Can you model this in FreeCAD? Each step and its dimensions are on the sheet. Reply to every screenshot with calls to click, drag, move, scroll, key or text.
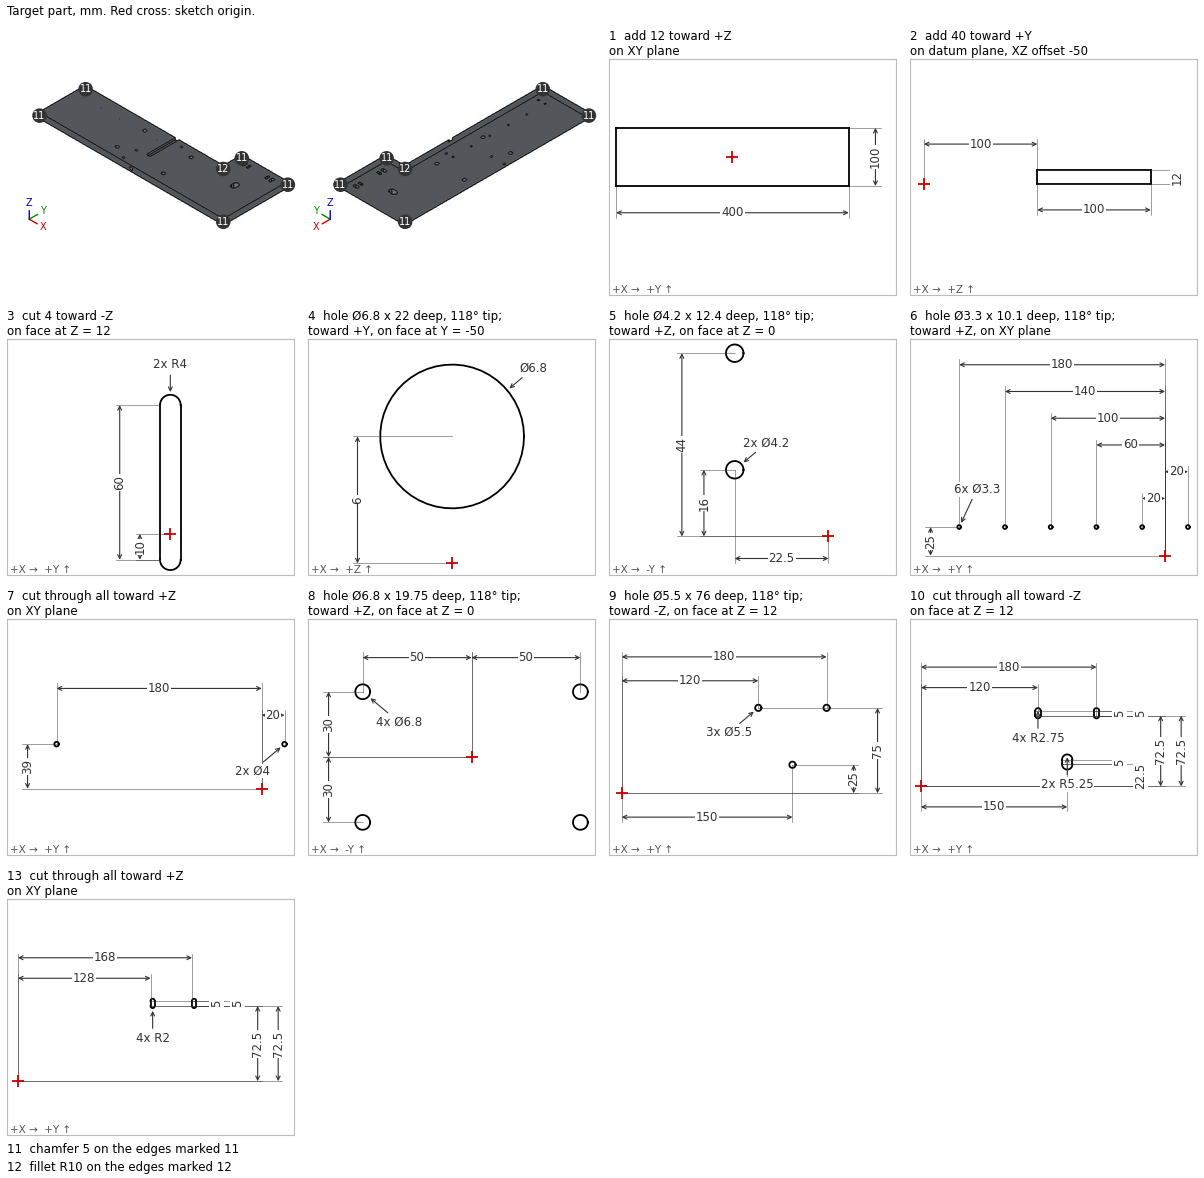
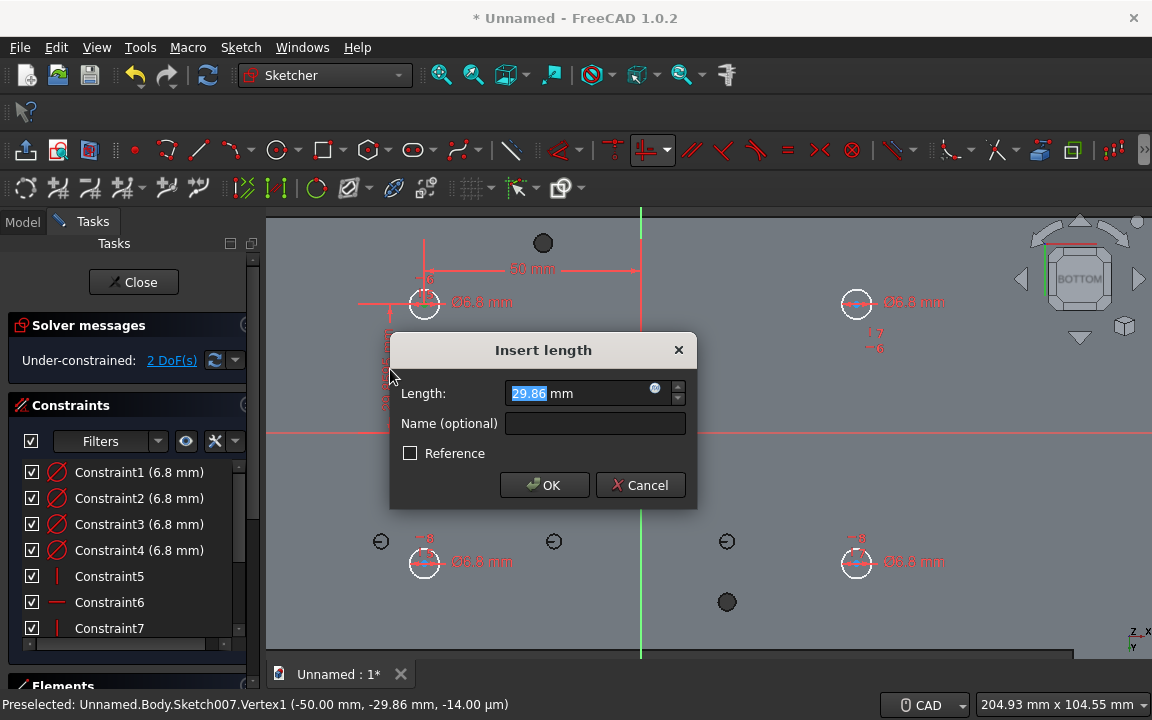
text(30)
key(Return)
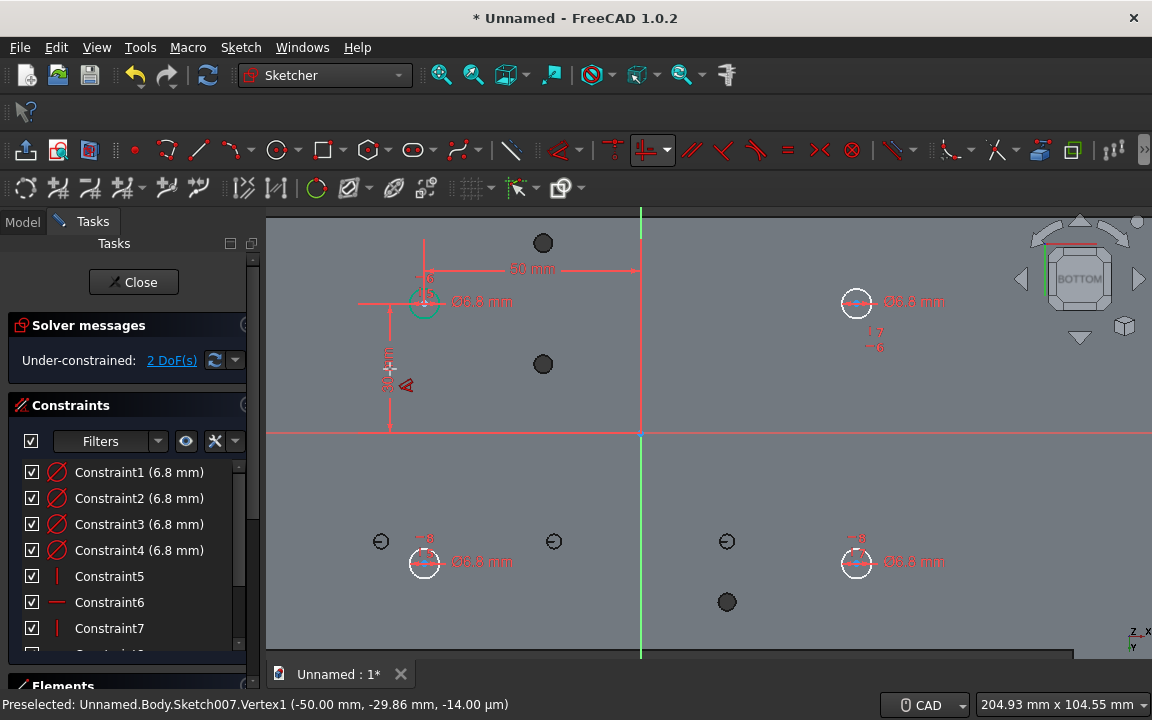
click(424, 564)
click(390, 499)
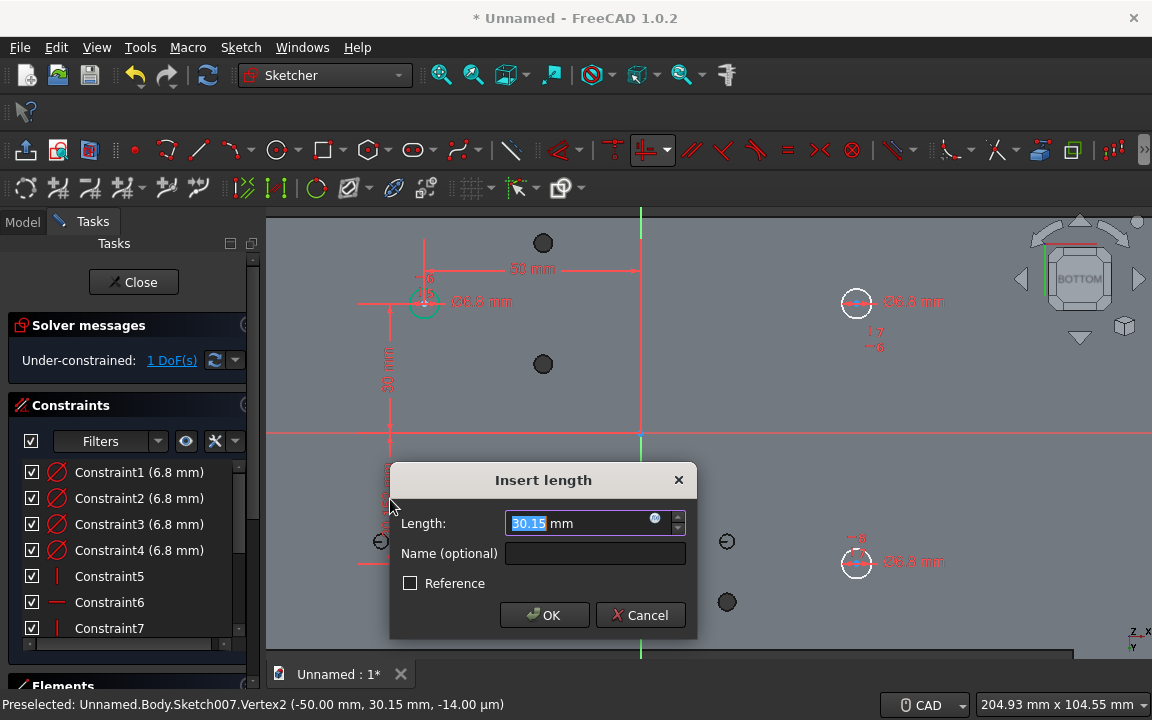
text(30)
key(Return)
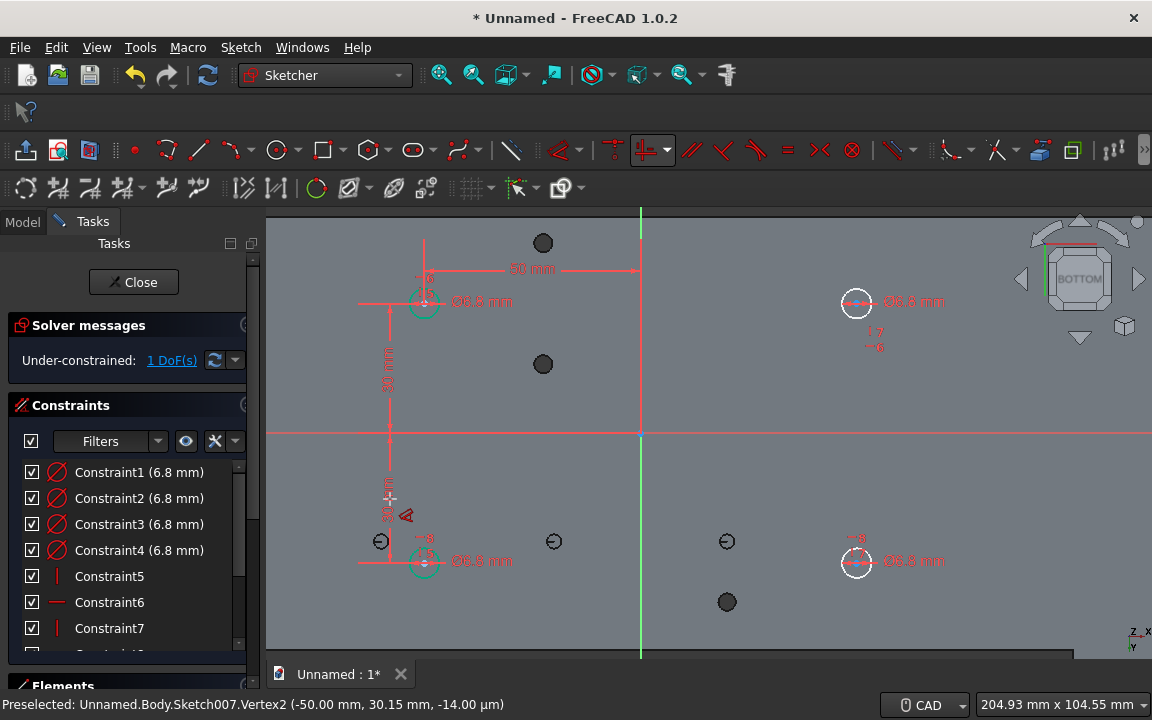
click(857, 304)
click(749, 270)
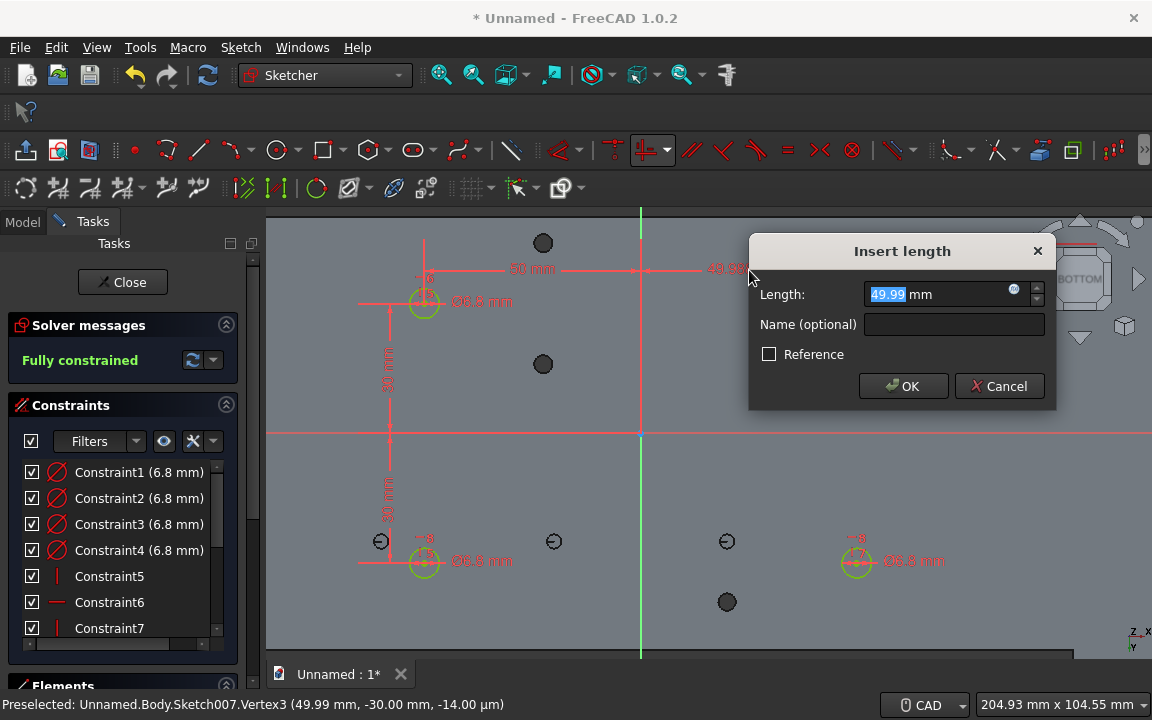
text(50)
key(Return)
key(Escape)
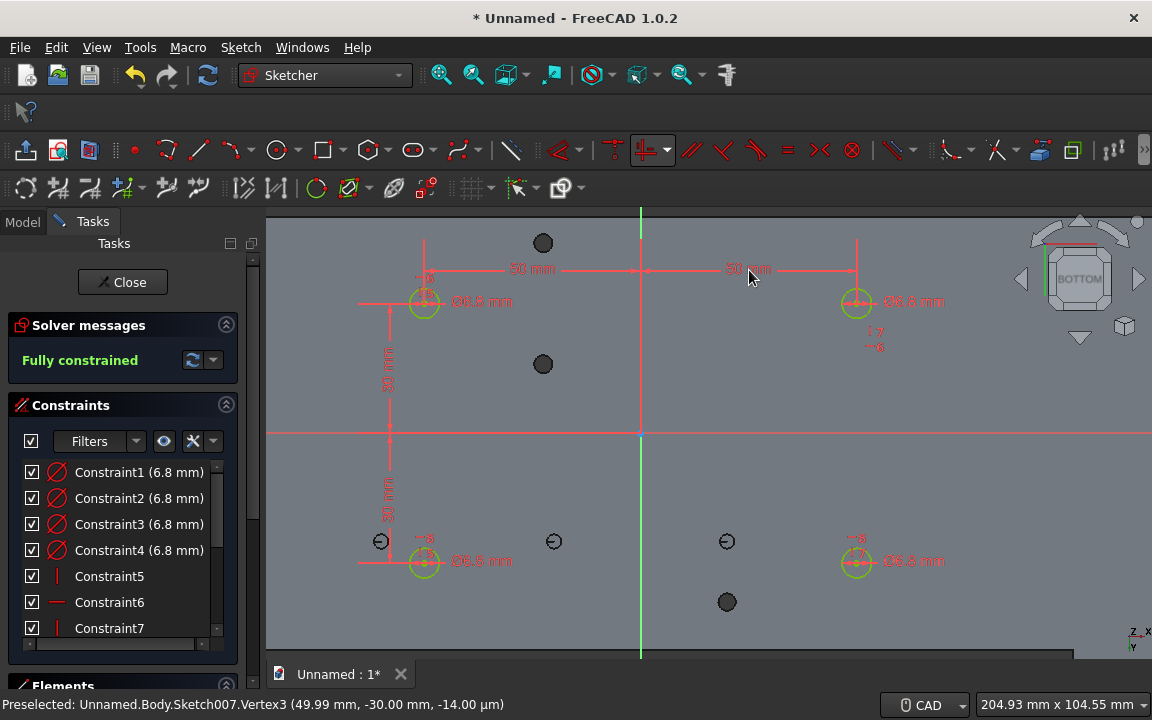
click(123, 282)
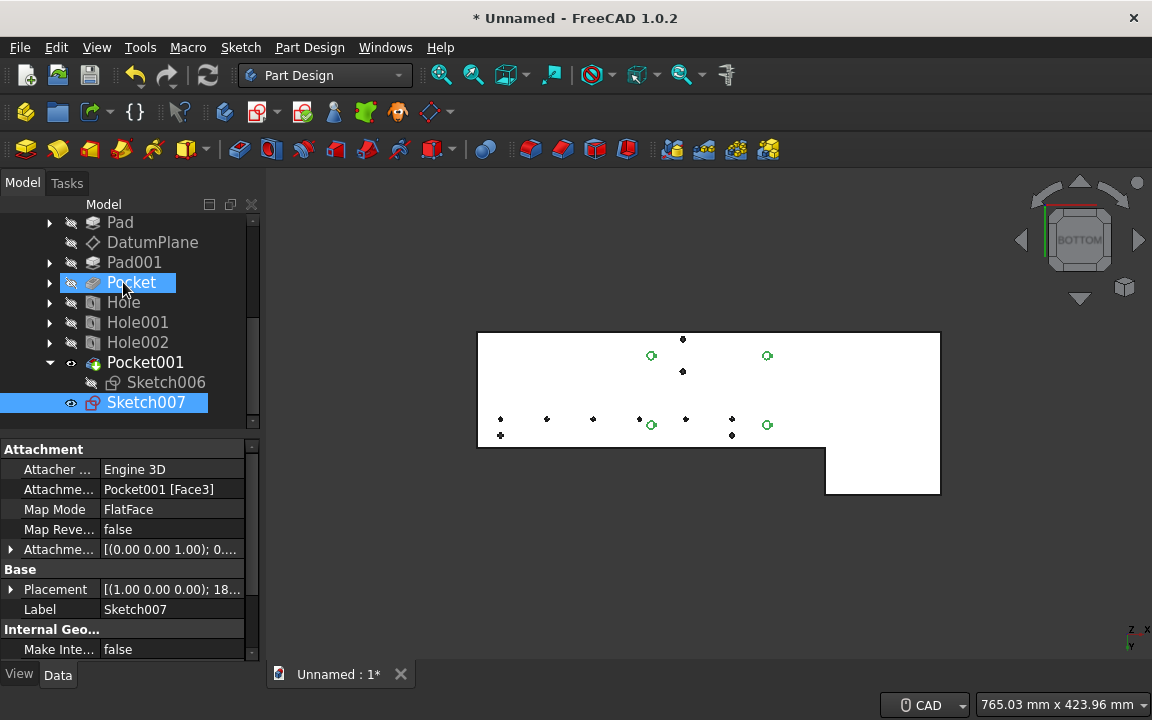
click(272, 150)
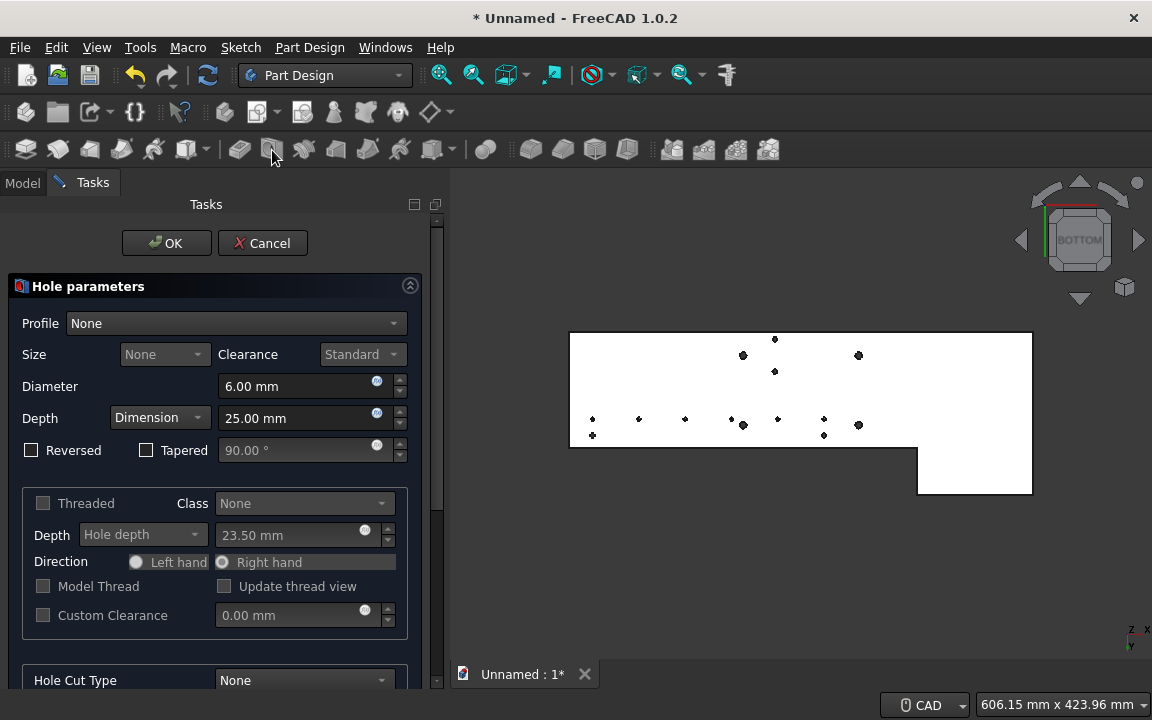
triple_click(305, 386)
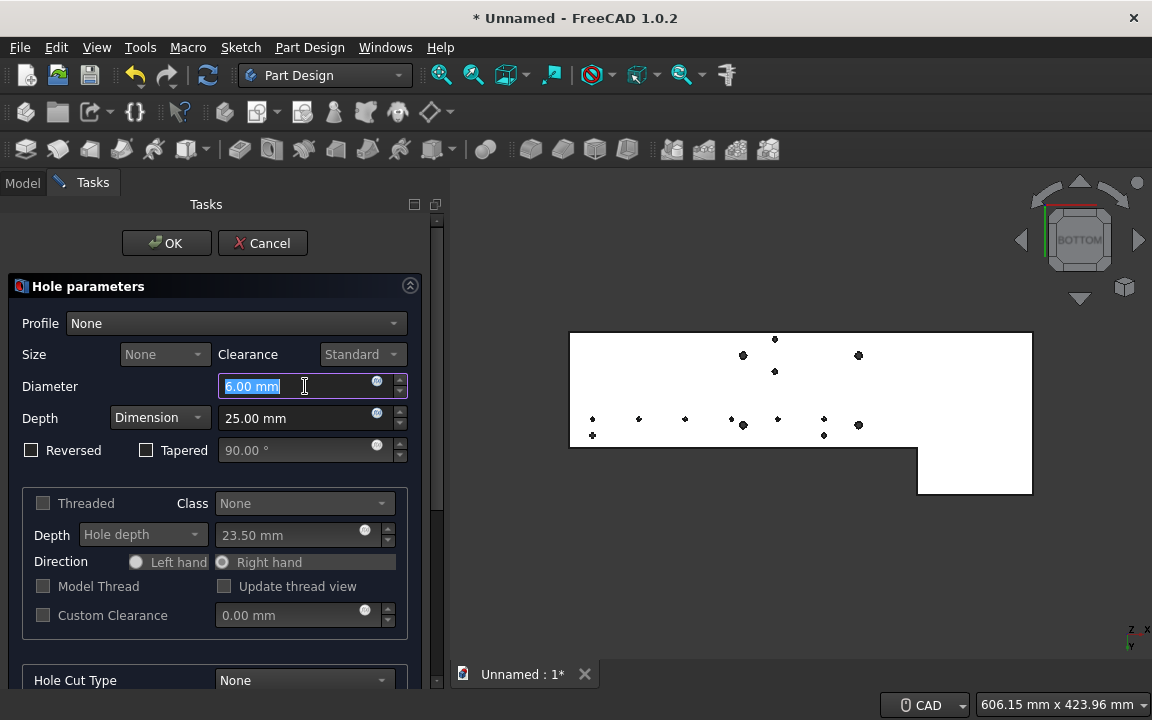
text(6.8)
key(Tab)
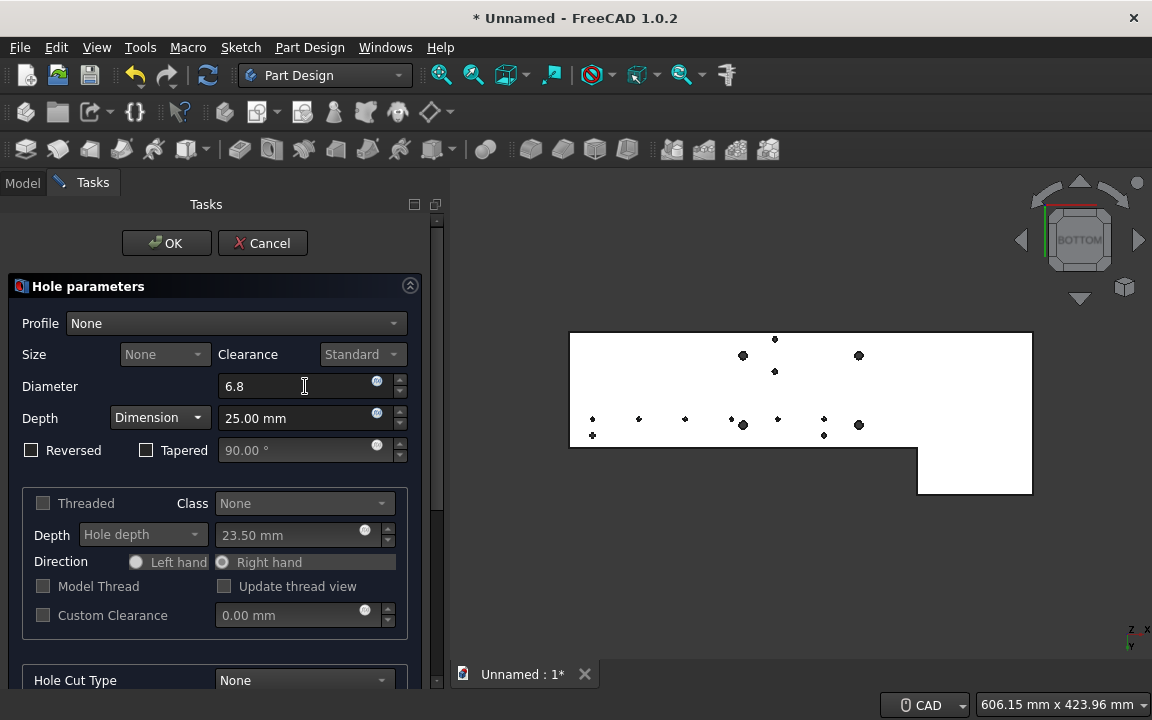
triple_click(305, 418)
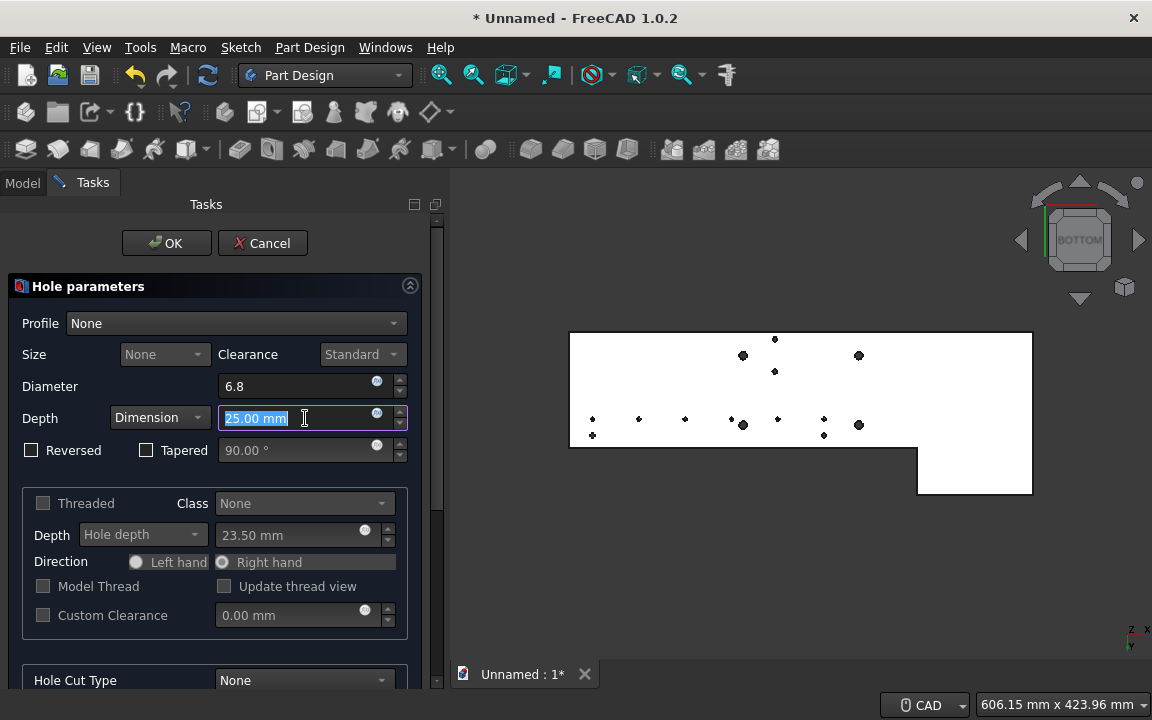
text(19.75)
key(Tab)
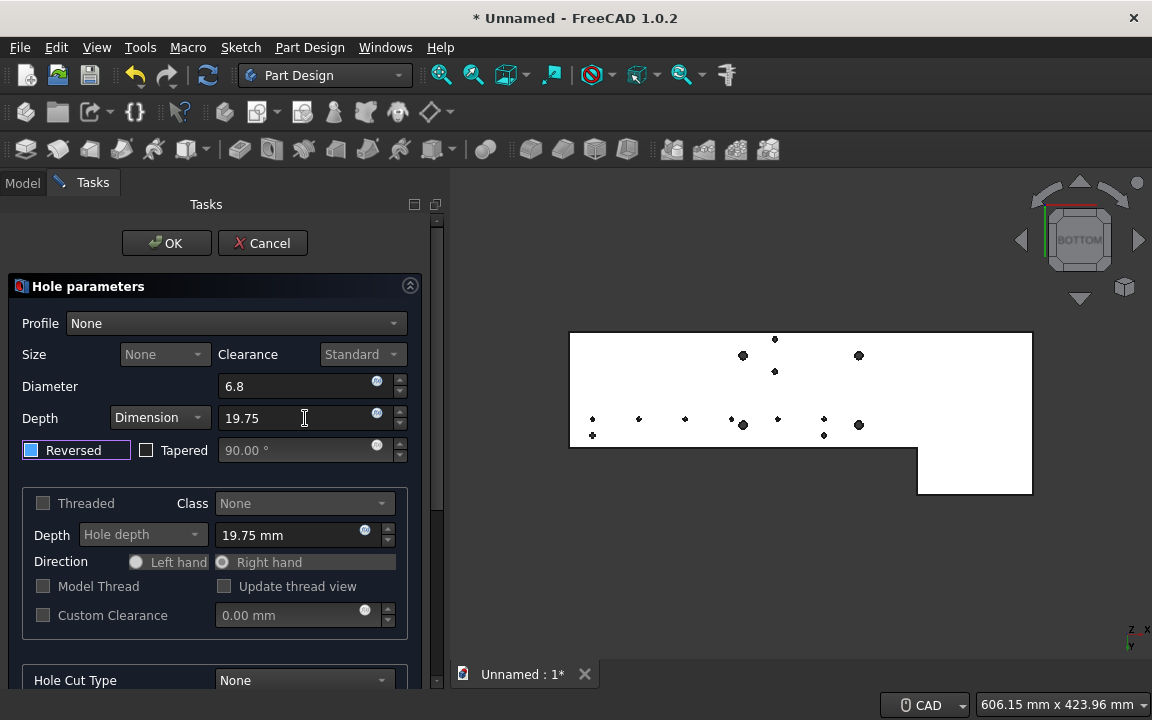
click(167, 243)